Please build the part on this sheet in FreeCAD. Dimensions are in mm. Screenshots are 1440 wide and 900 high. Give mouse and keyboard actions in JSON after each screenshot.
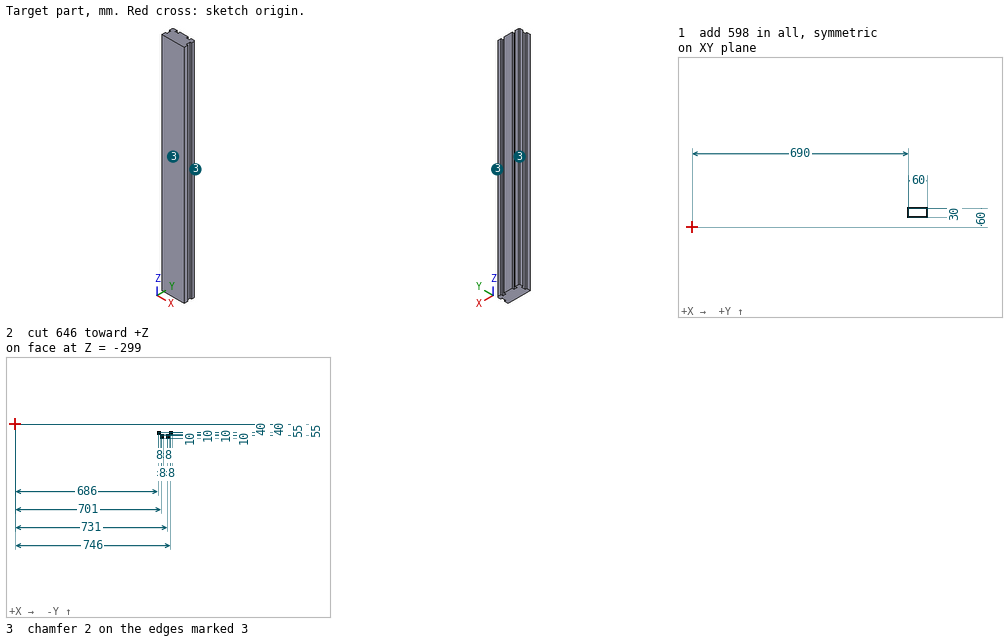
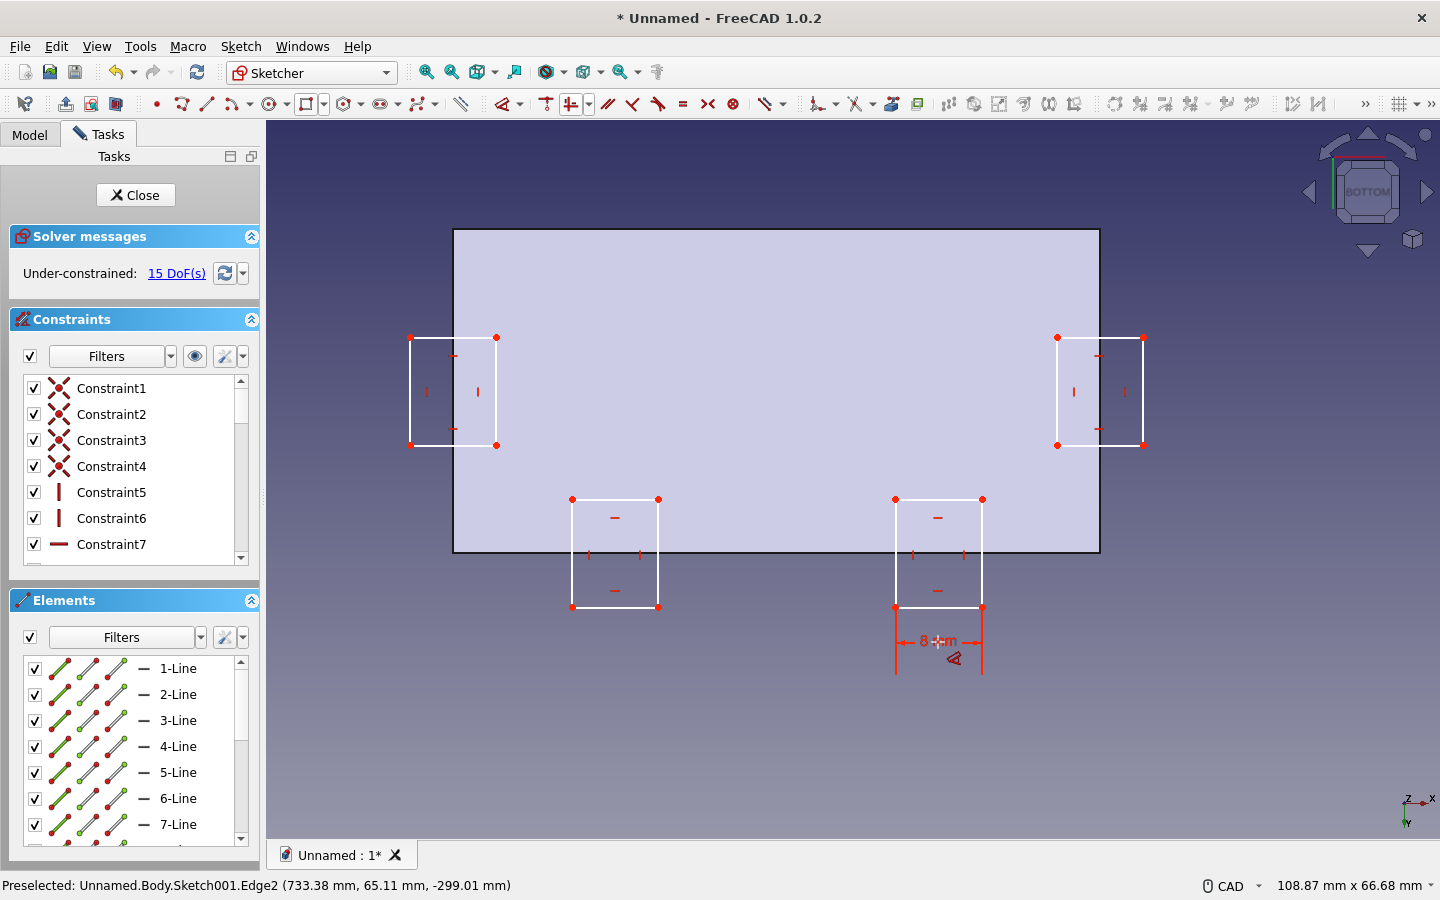
{"action": "left_click", "coordinate": [1083, 446]}
{"action": "left_click", "coordinate": [1100, 412]}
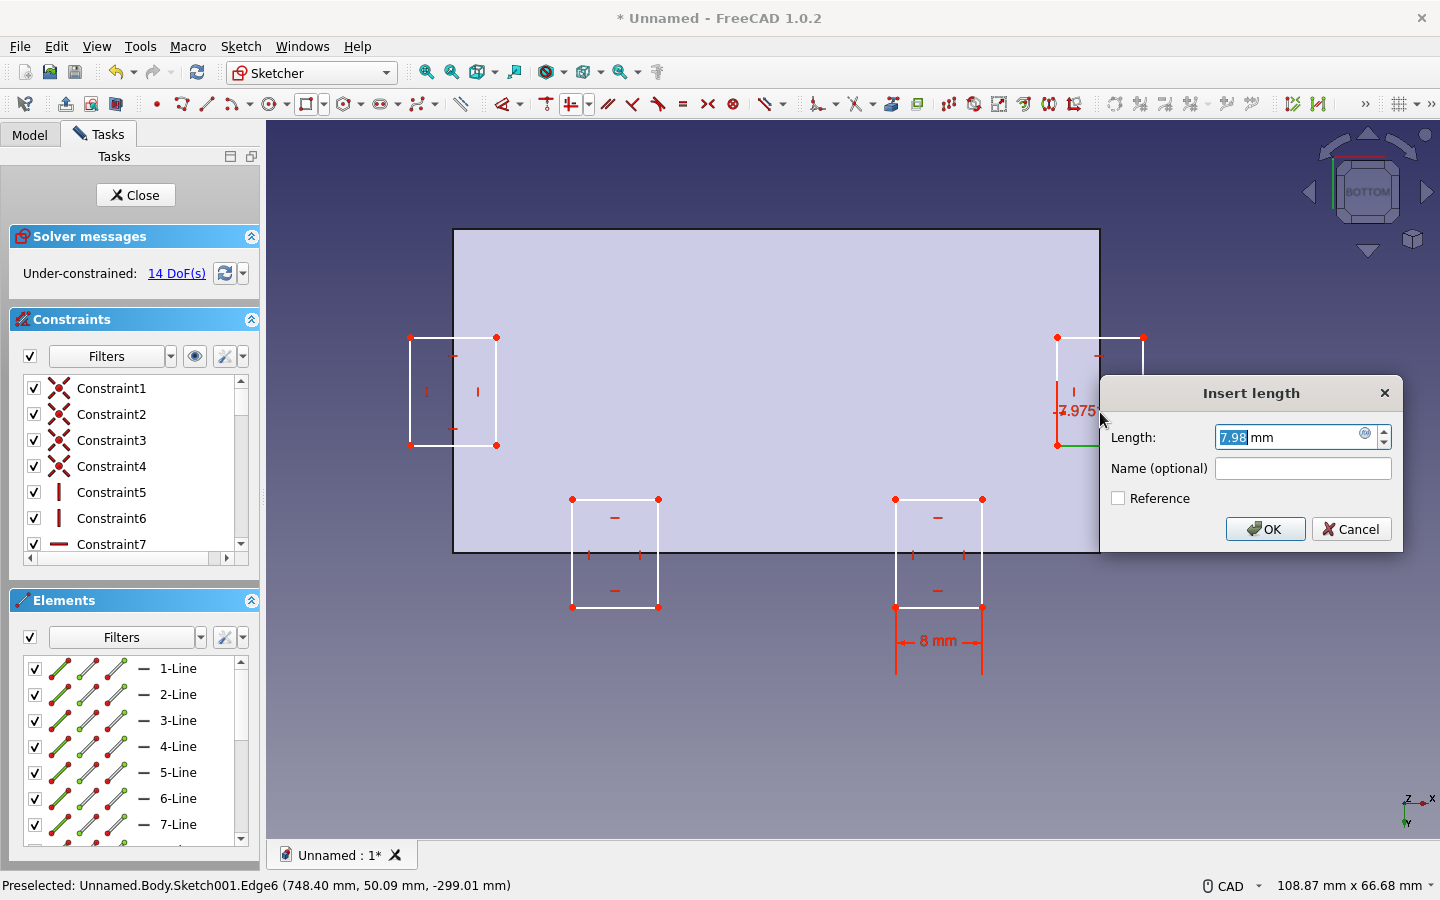
{"action": "type", "text": "8"}
{"action": "key", "text": "Return"}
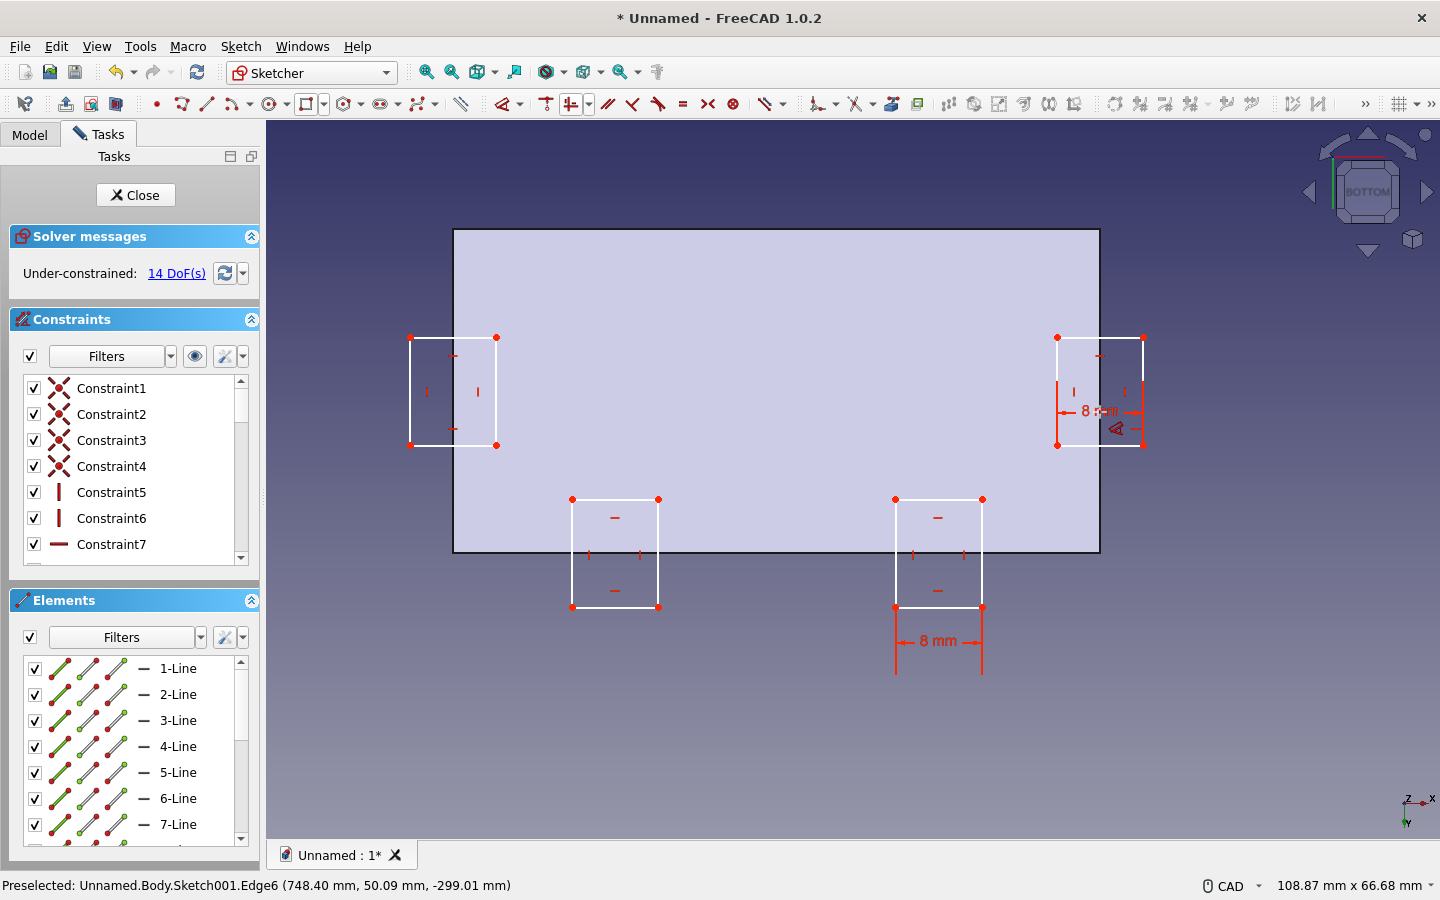
{"action": "left_click", "coordinate": [436, 446]}
{"action": "left_click", "coordinate": [453, 412]}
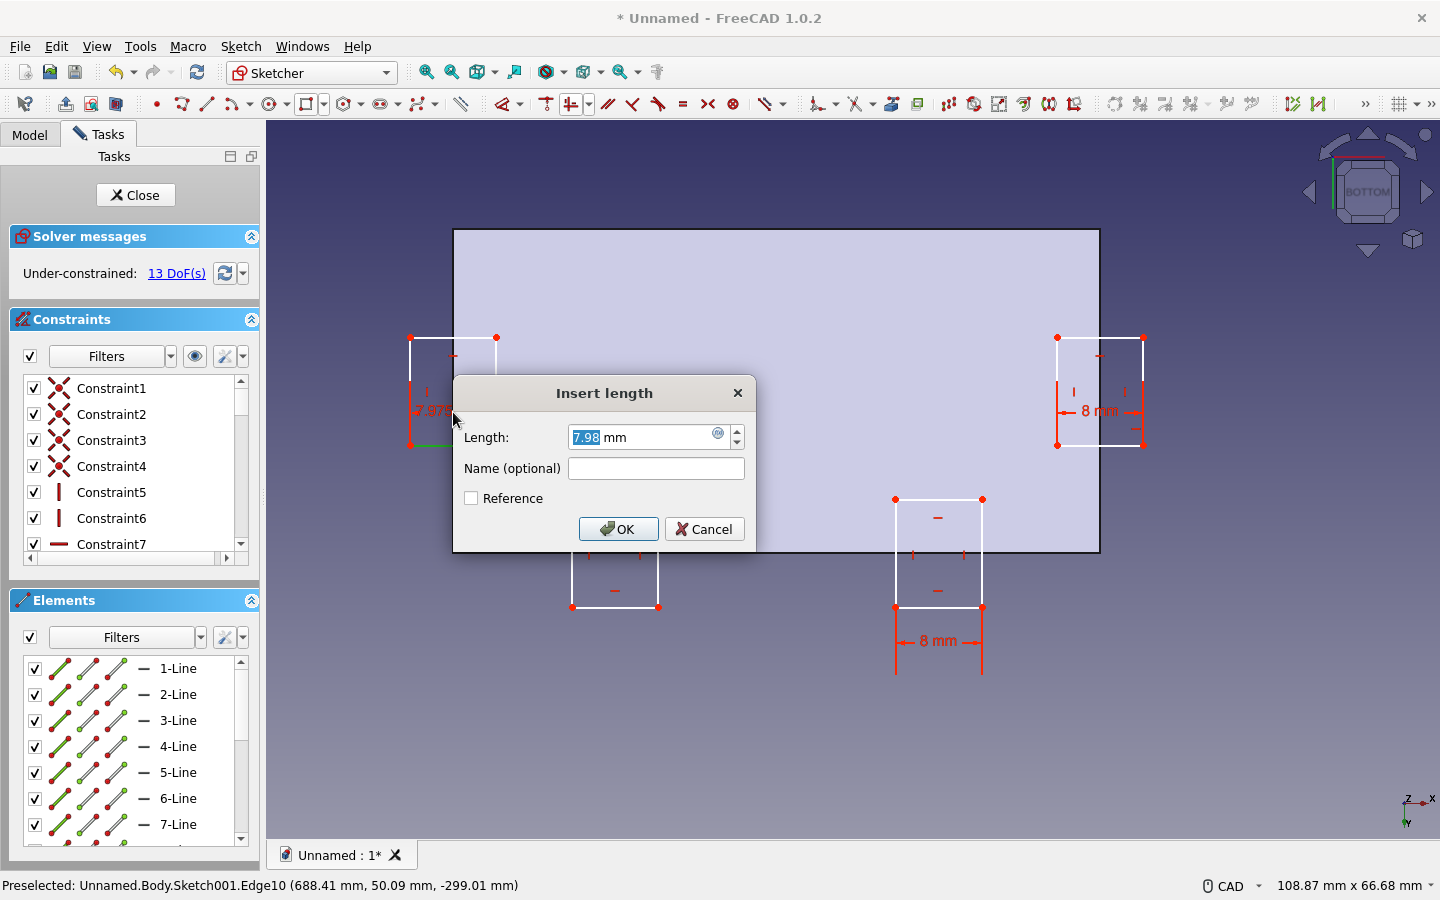
{"action": "type", "text": "8"}
{"action": "key", "text": "Return"}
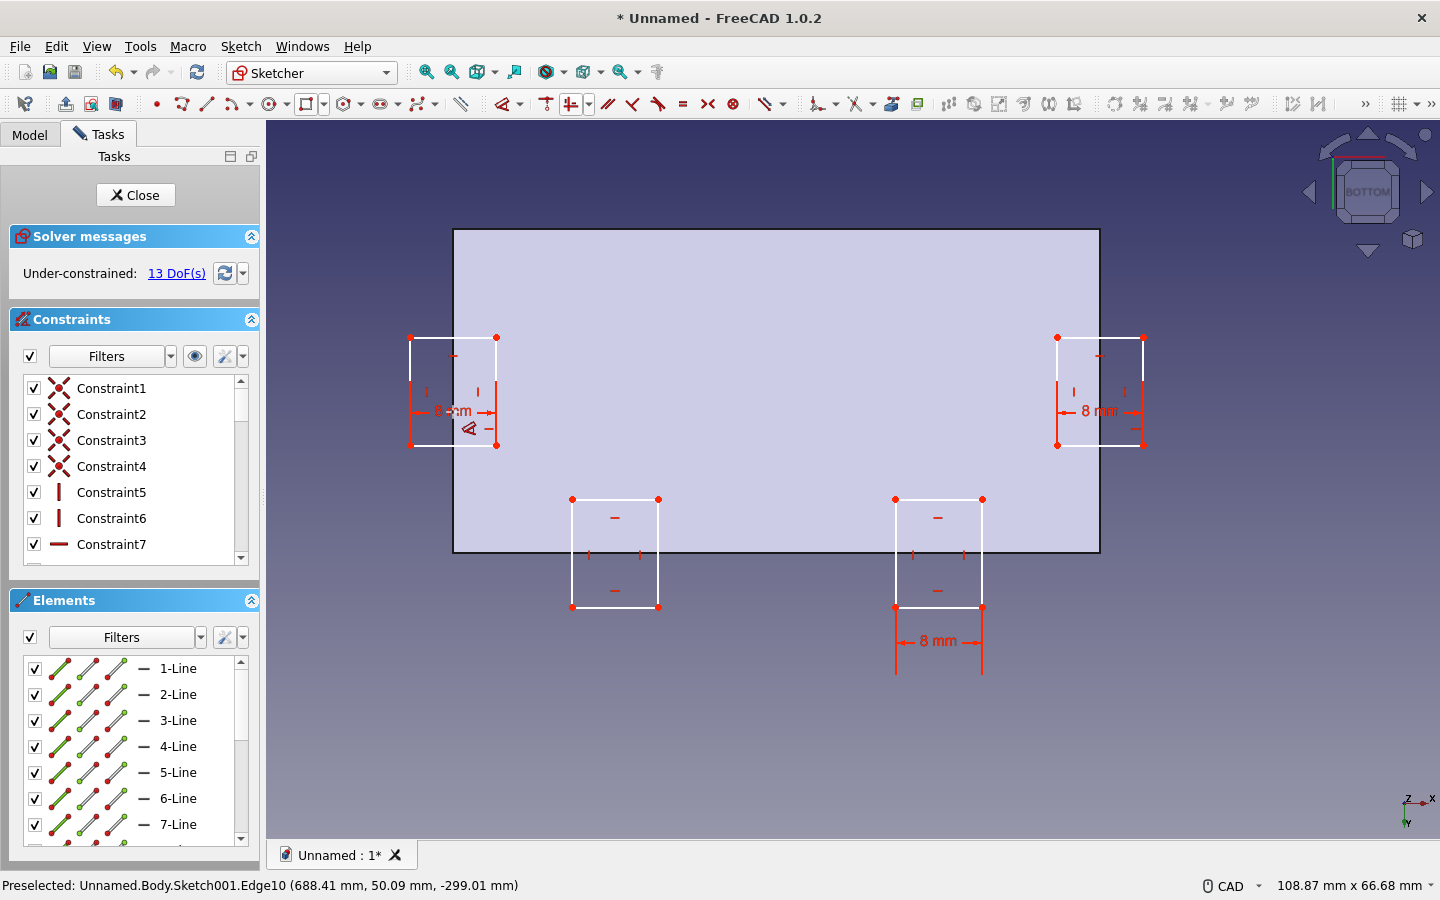
{"action": "left_click", "coordinate": [598, 608]}
{"action": "left_click", "coordinate": [615, 642]}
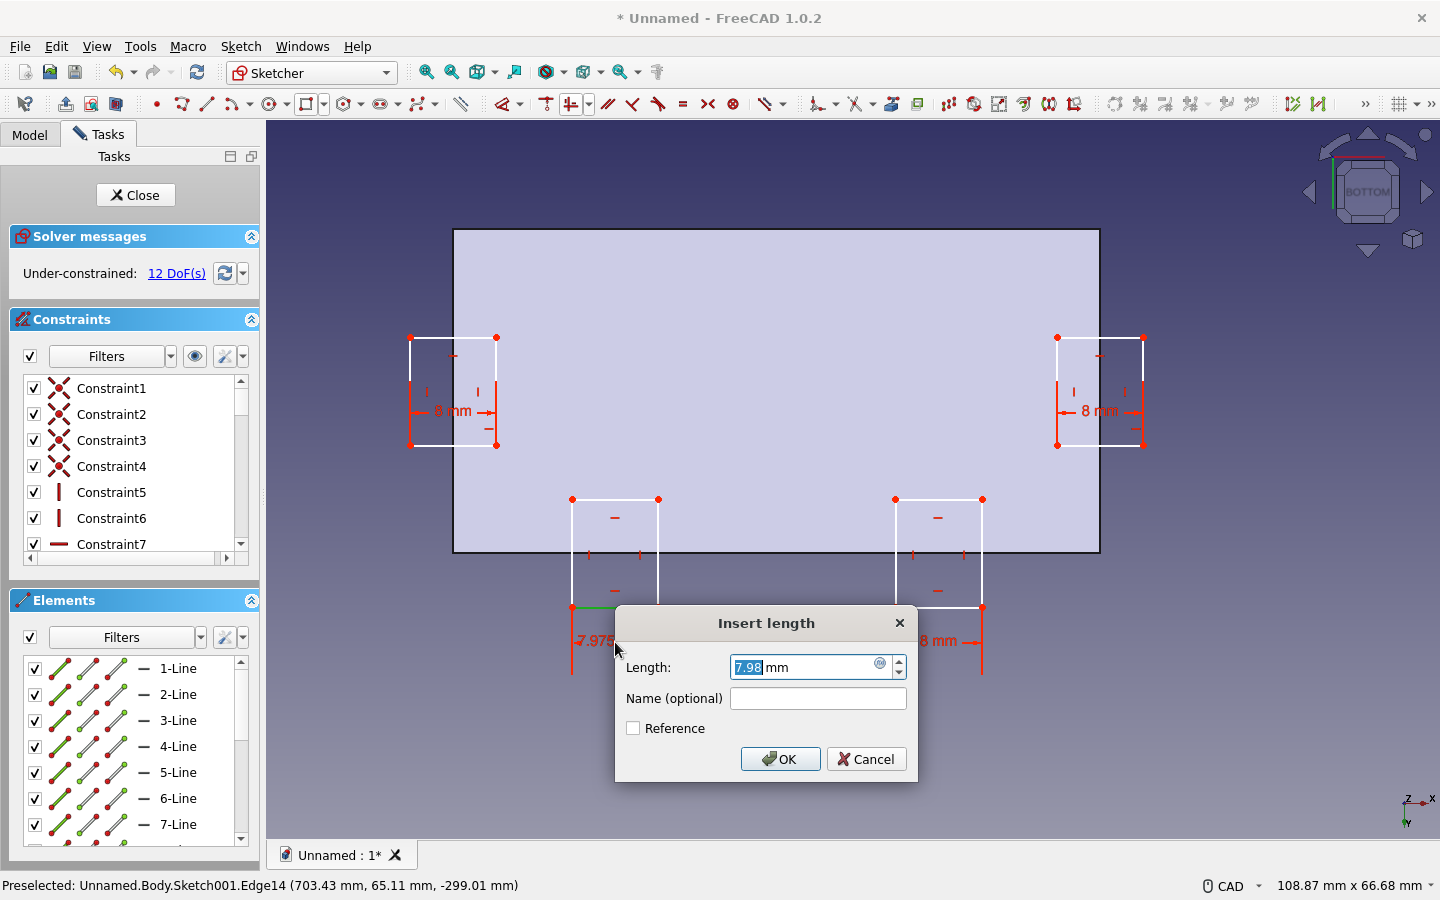
{"action": "type", "text": "8"}
{"action": "key", "text": "Return"}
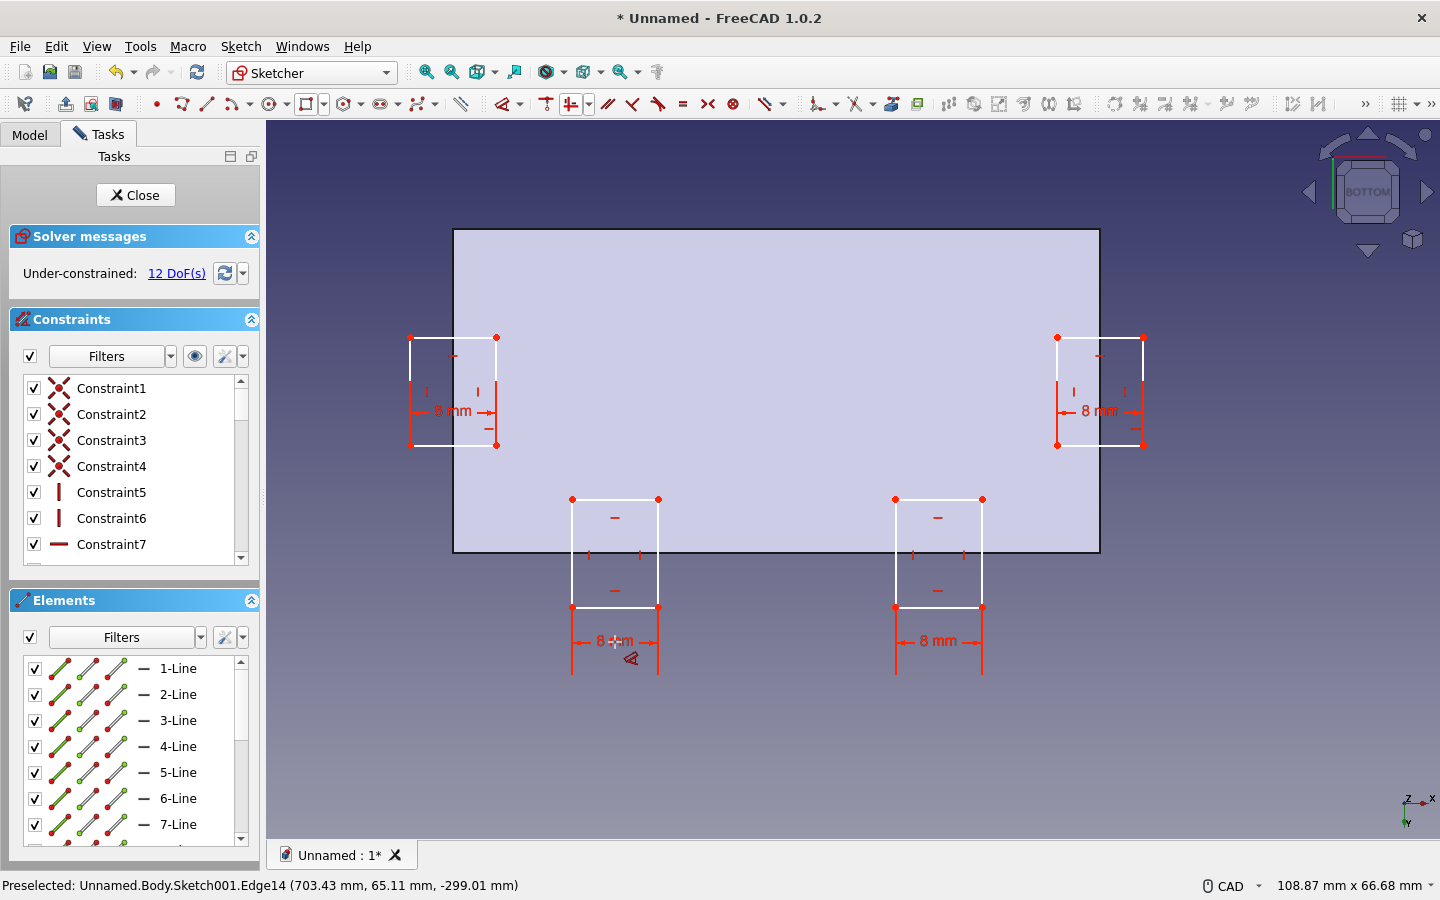
{"action": "left_click", "coordinate": [896, 532]}
{"action": "left_click", "coordinate": [930, 554]}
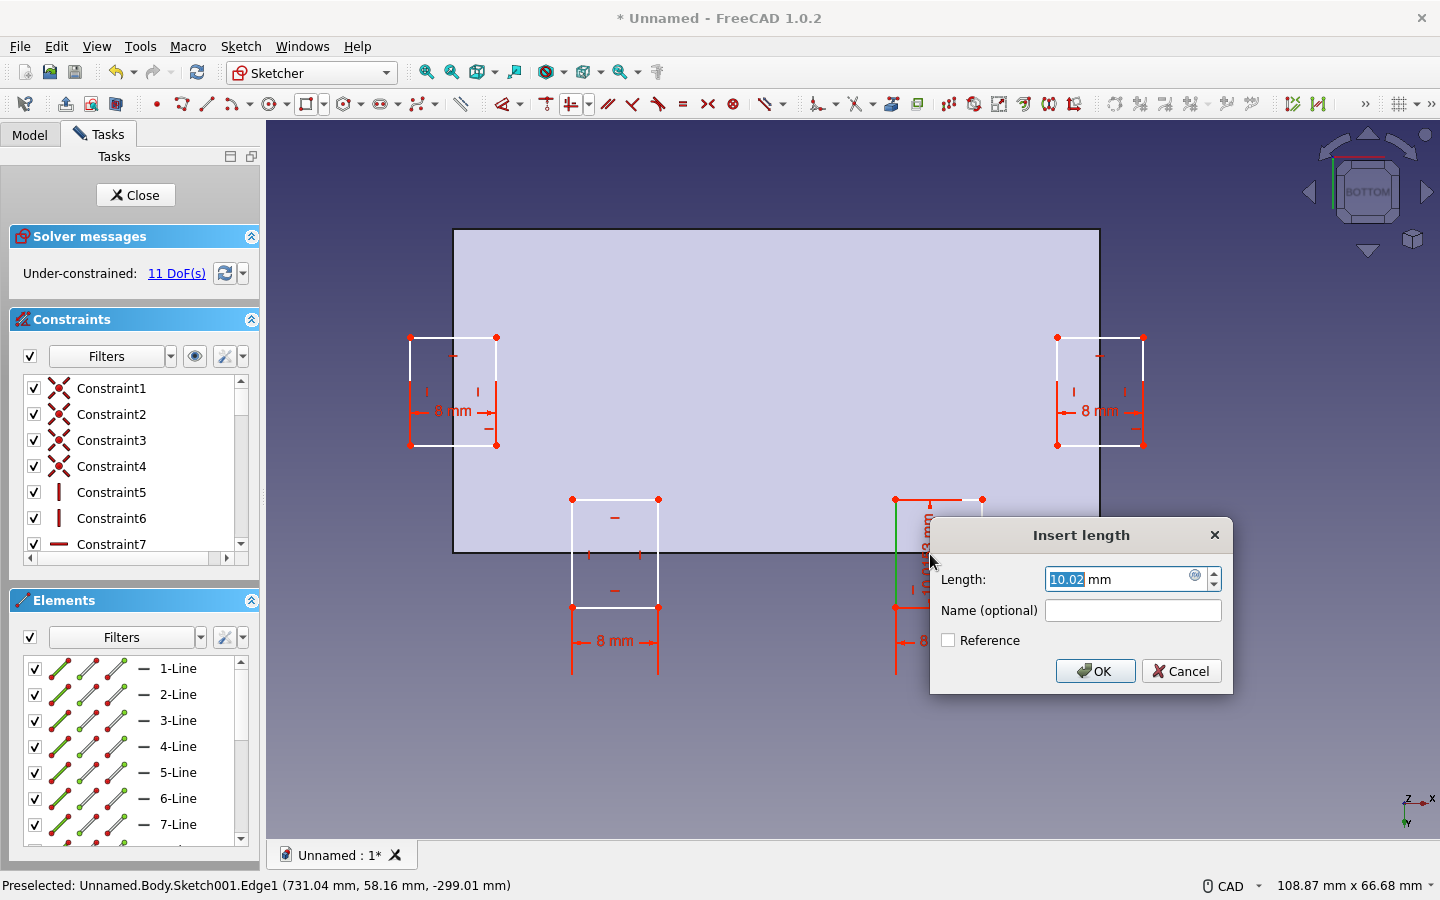
{"action": "type", "text": "10"}
{"action": "key", "text": "Return"}